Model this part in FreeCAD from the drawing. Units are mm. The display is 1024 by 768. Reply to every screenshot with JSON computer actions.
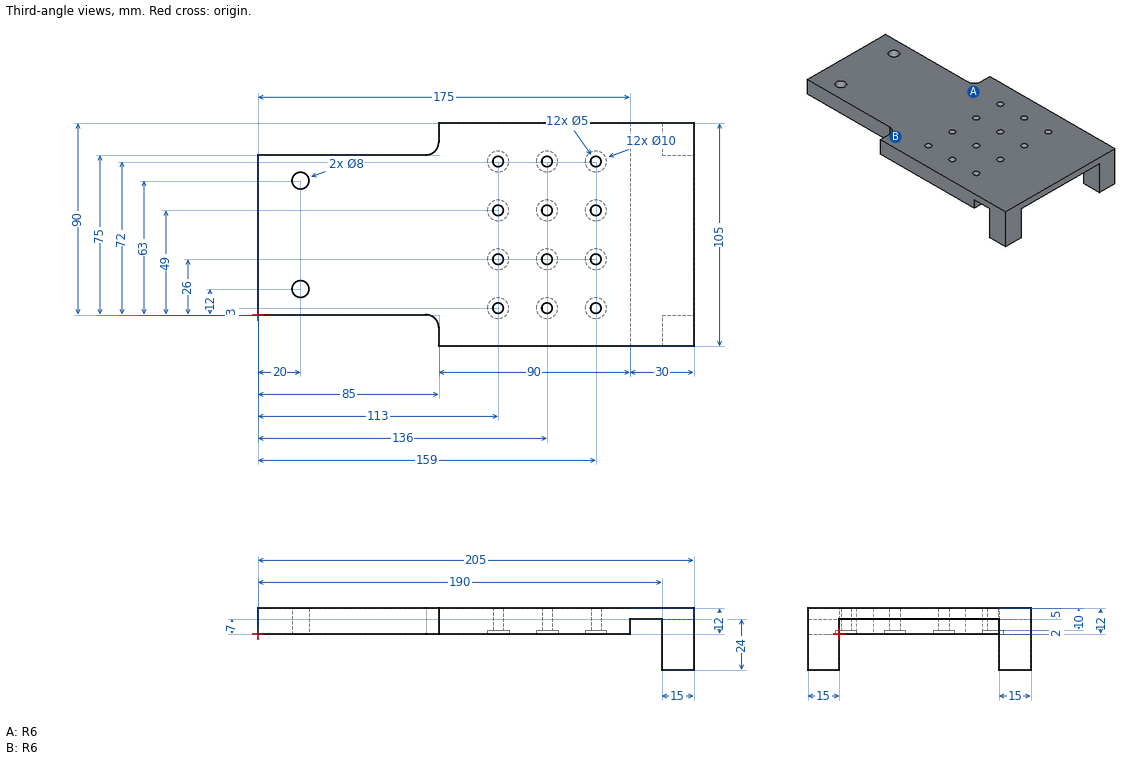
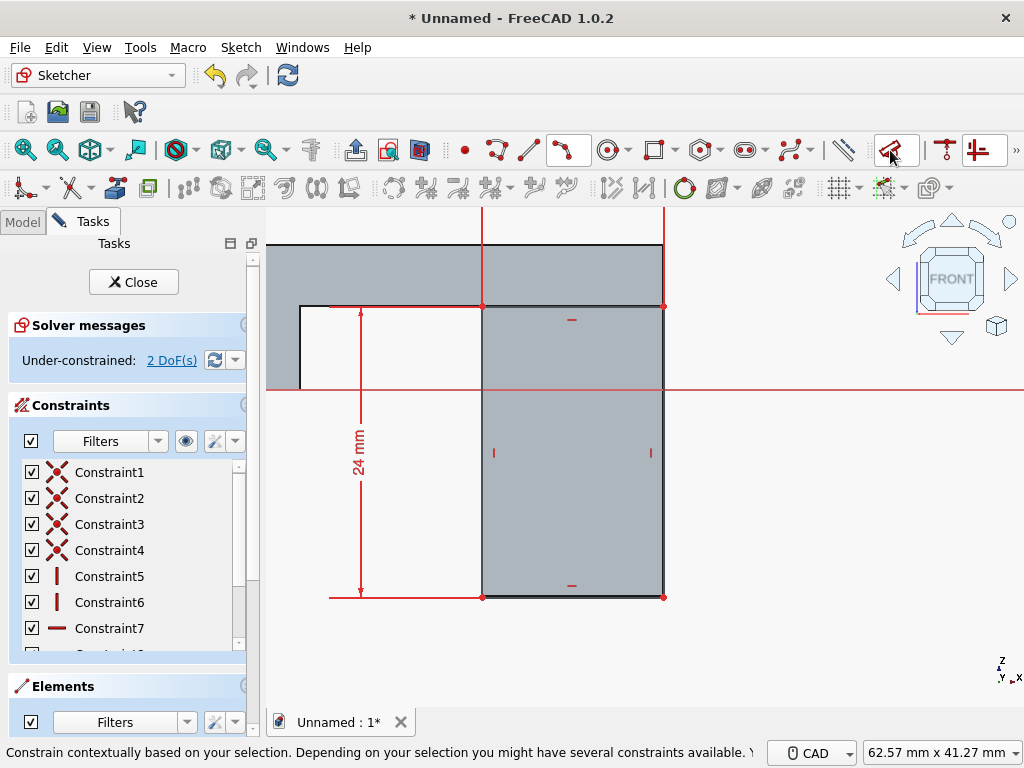
{"action": "left_click", "coordinate": [482, 307]}
{"action": "left_click", "coordinate": [516, 349]}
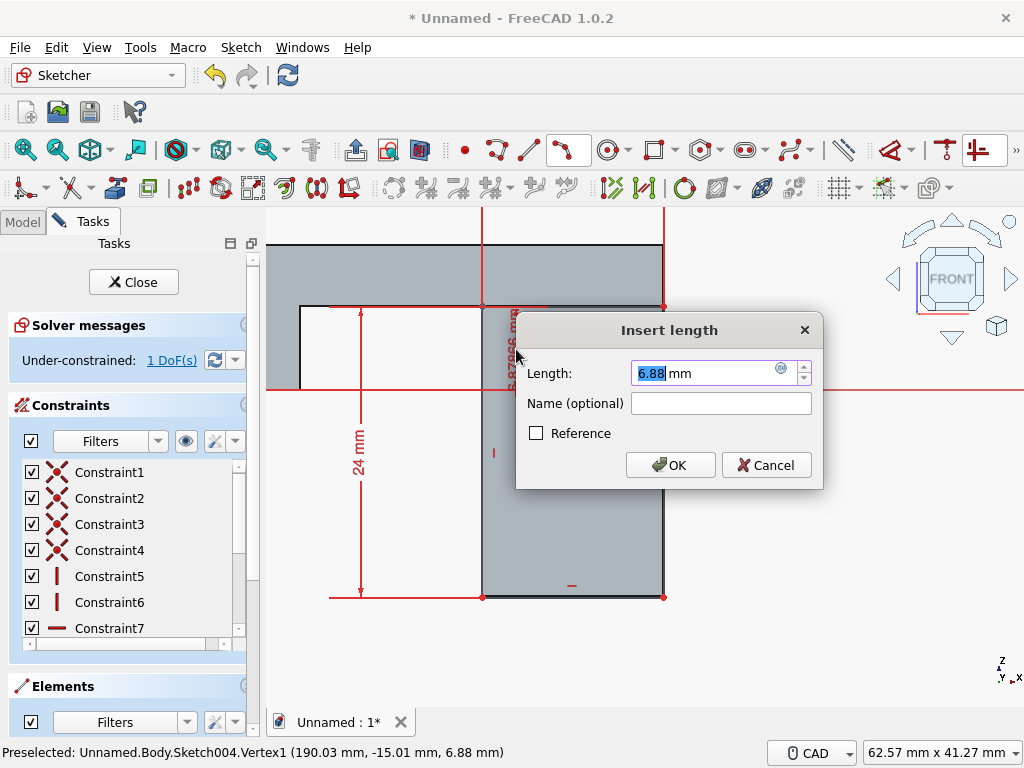
{"action": "type", "text": "7"}
{"action": "key", "text": "Return"}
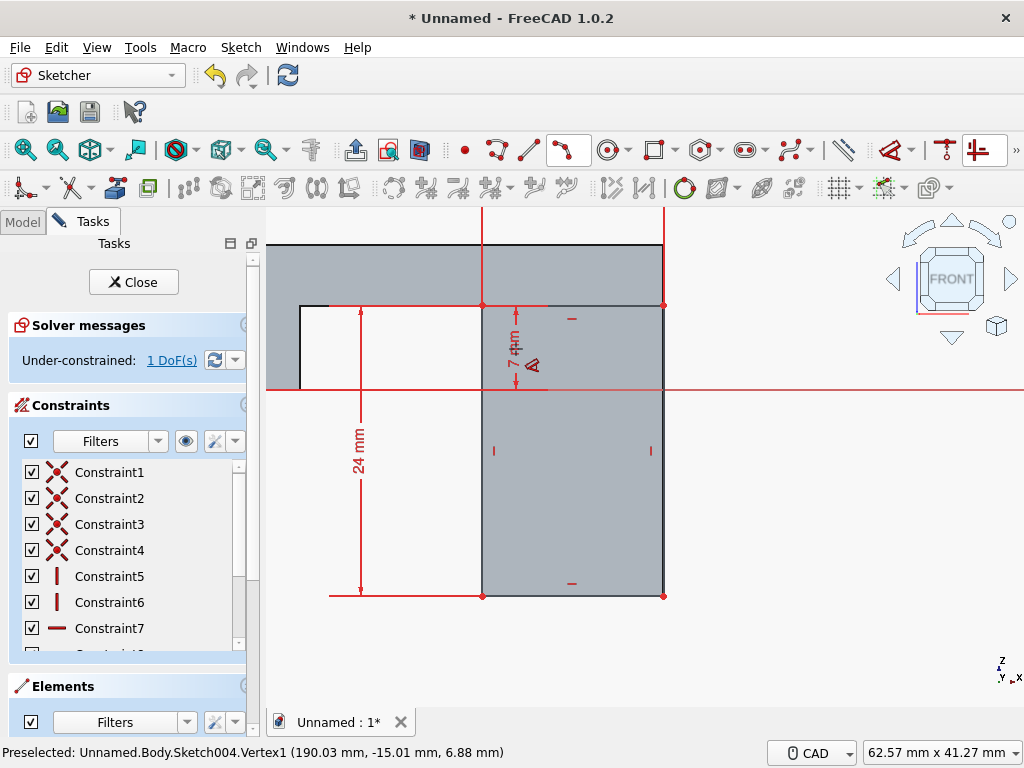
{"action": "left_click", "coordinate": [482, 306]}
{"action": "left_click", "coordinate": [388, 272]}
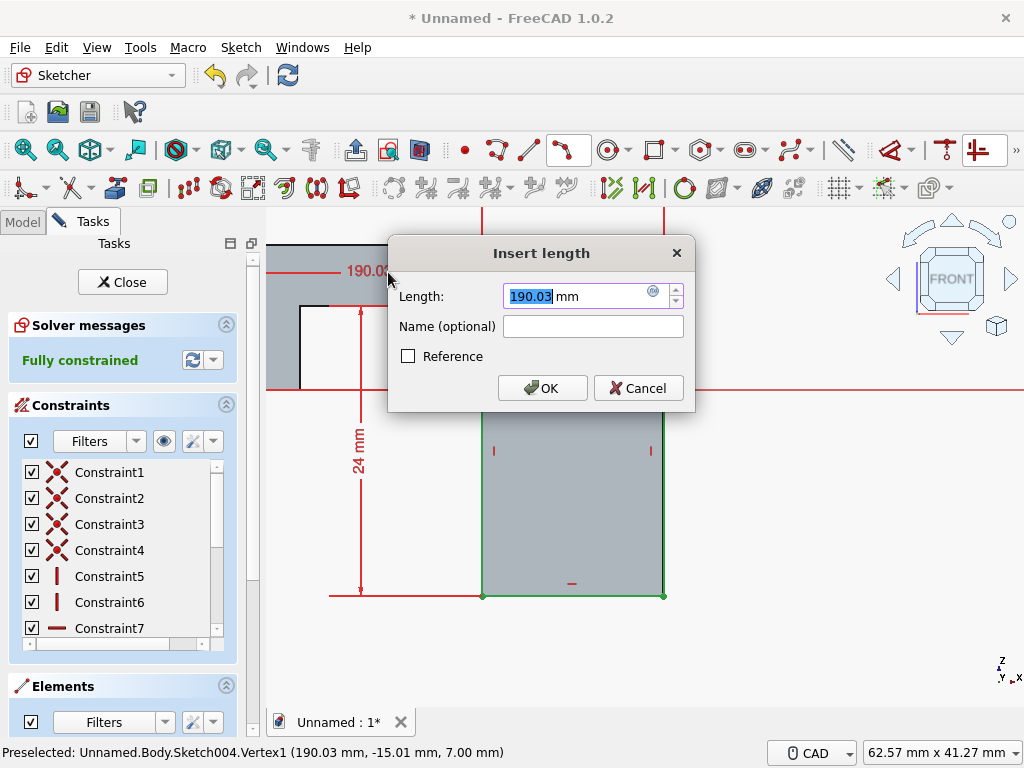
{"action": "type", "text": "190"}
{"action": "key", "text": "Return"}
{"action": "key", "text": "Escape"}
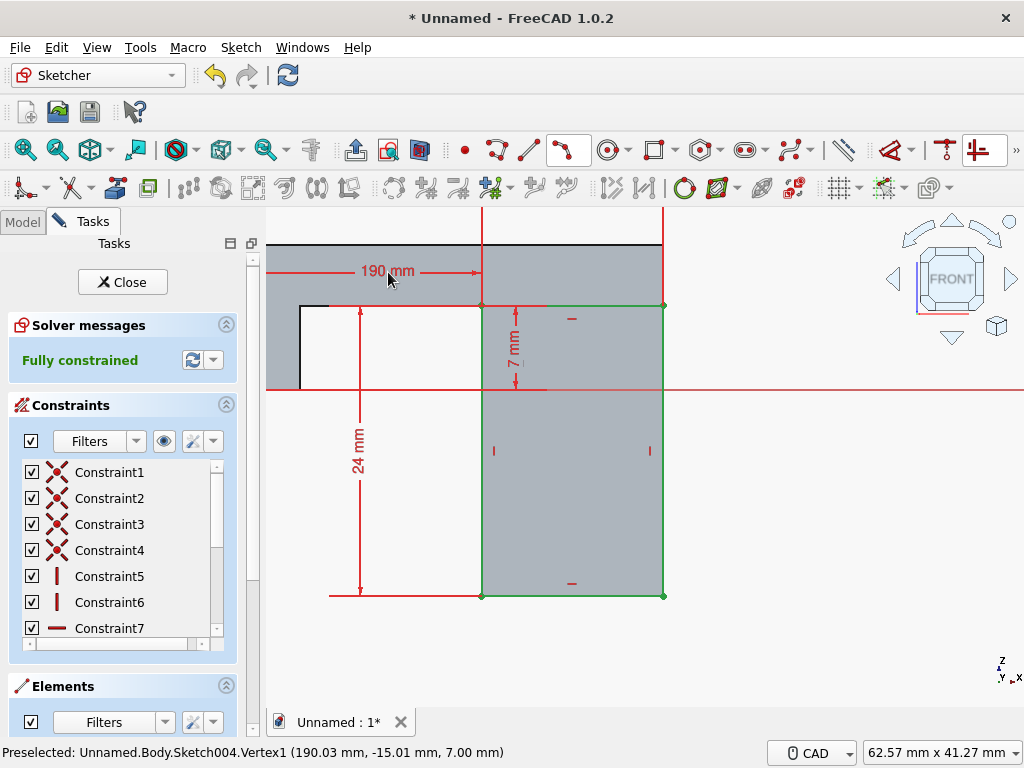
{"action": "left_click", "coordinate": [123, 282]}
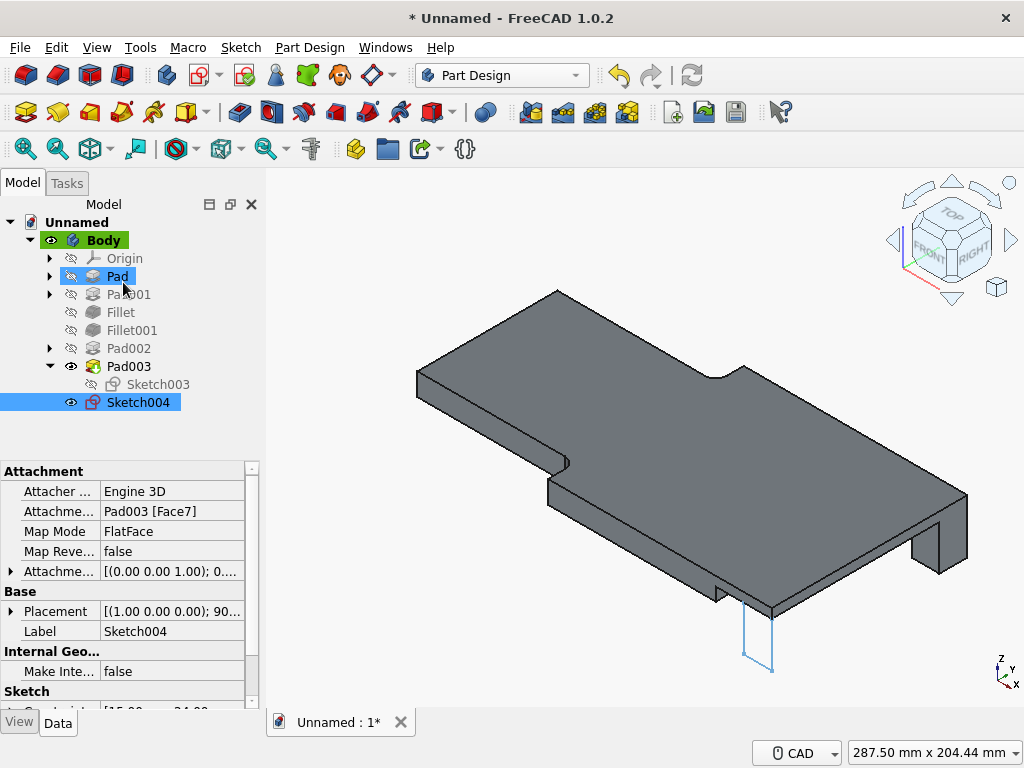
{"action": "left_click", "coordinate": [26, 112]}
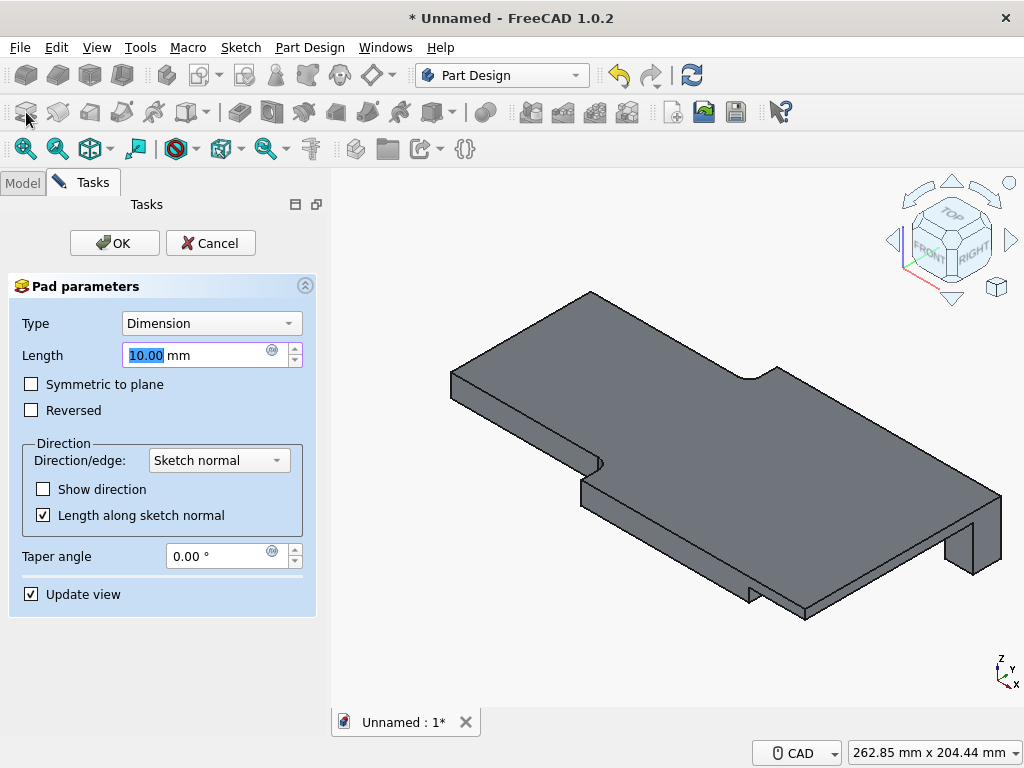
{"action": "type", "text": "15"}
{"action": "key", "text": "Tab"}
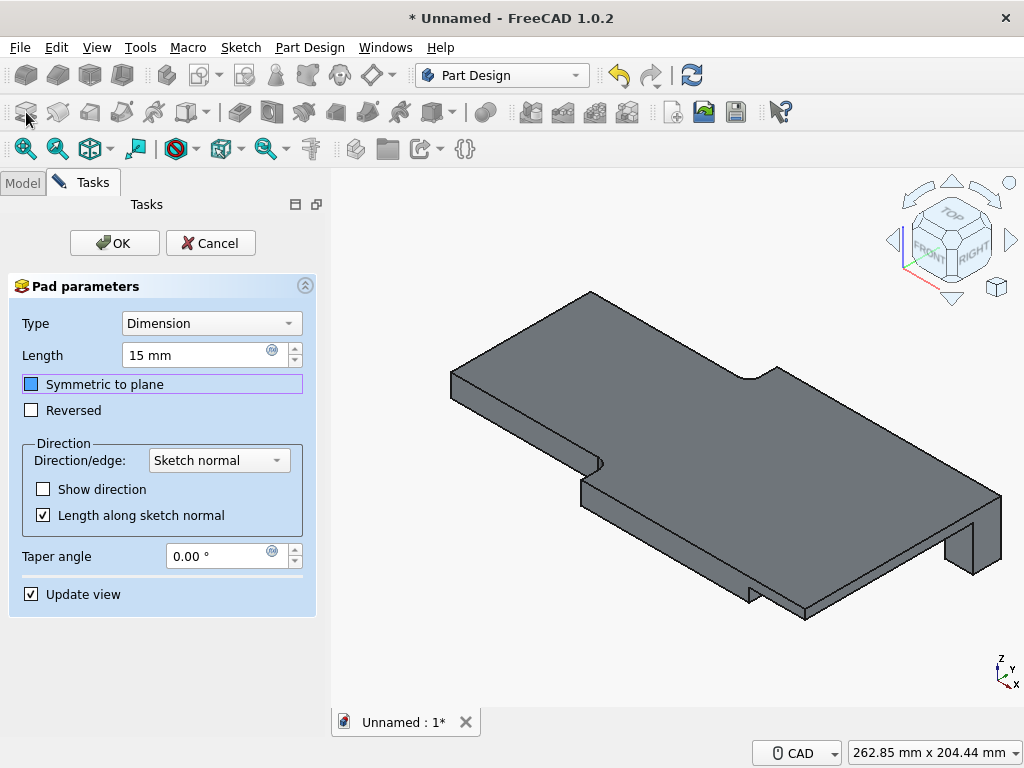
{"action": "left_click", "coordinate": [30, 410]}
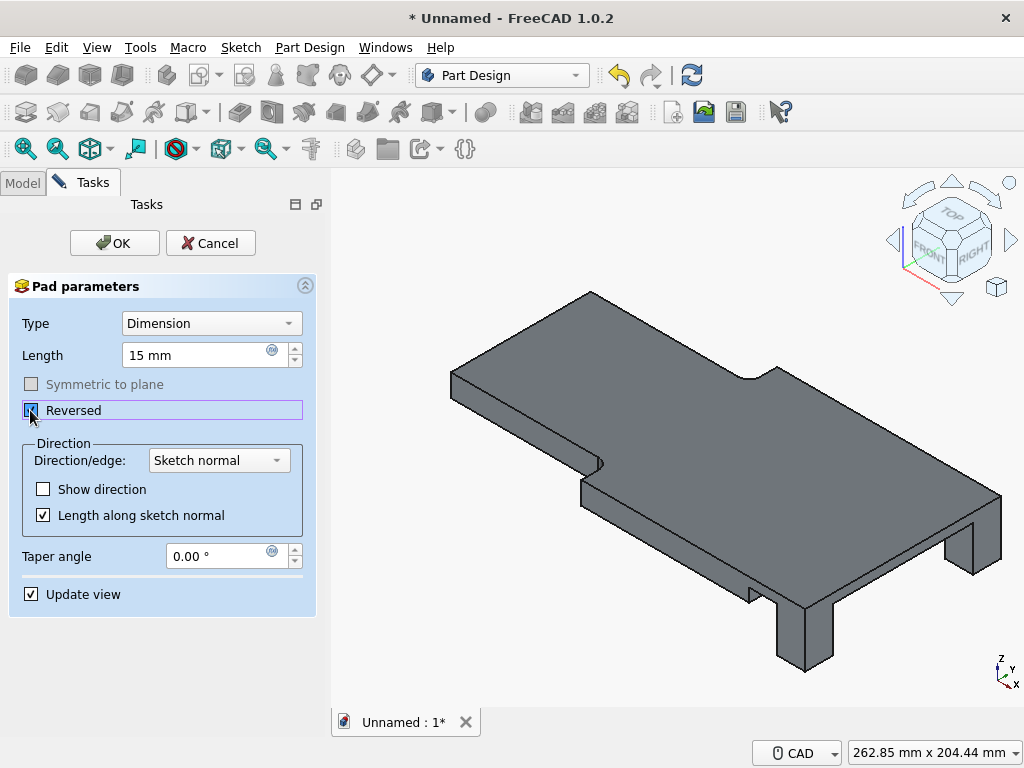
{"action": "left_click", "coordinate": [115, 243]}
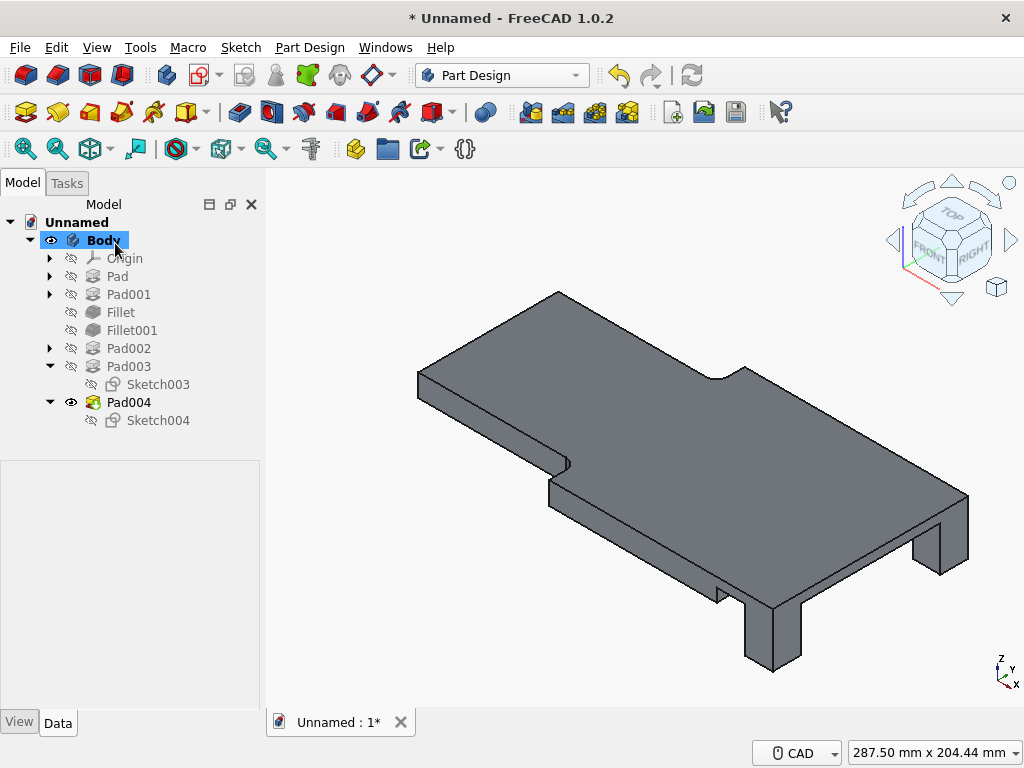
{"action": "left_click", "coordinate": [200, 76]}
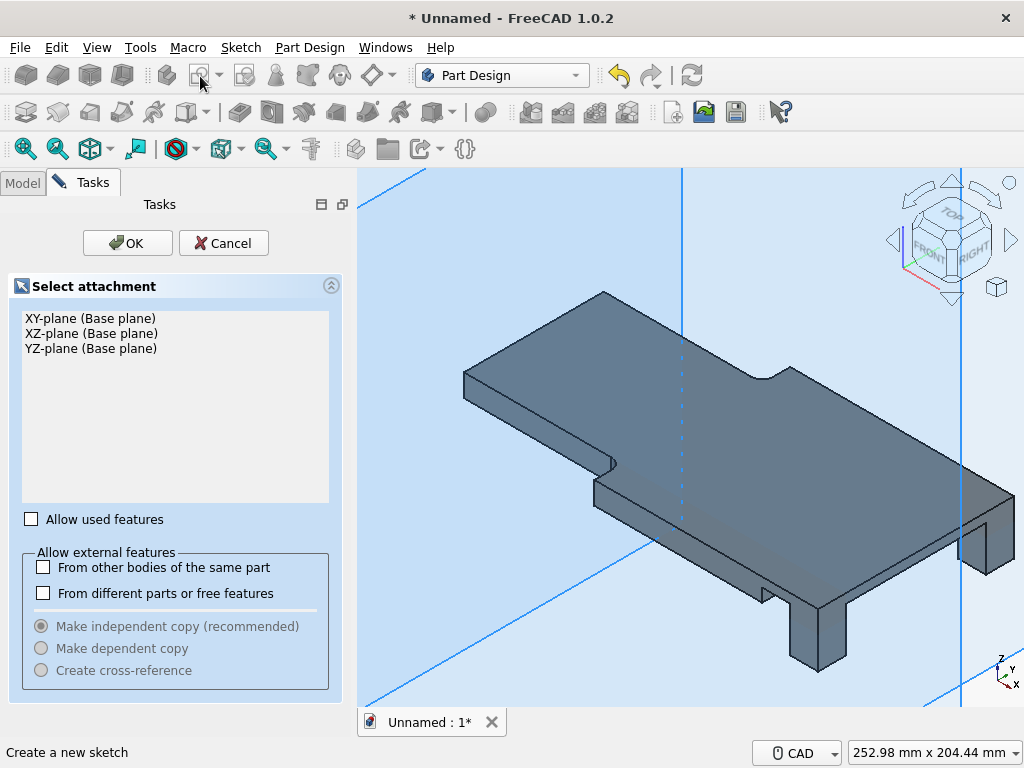
{"action": "left_click", "coordinate": [82, 318]}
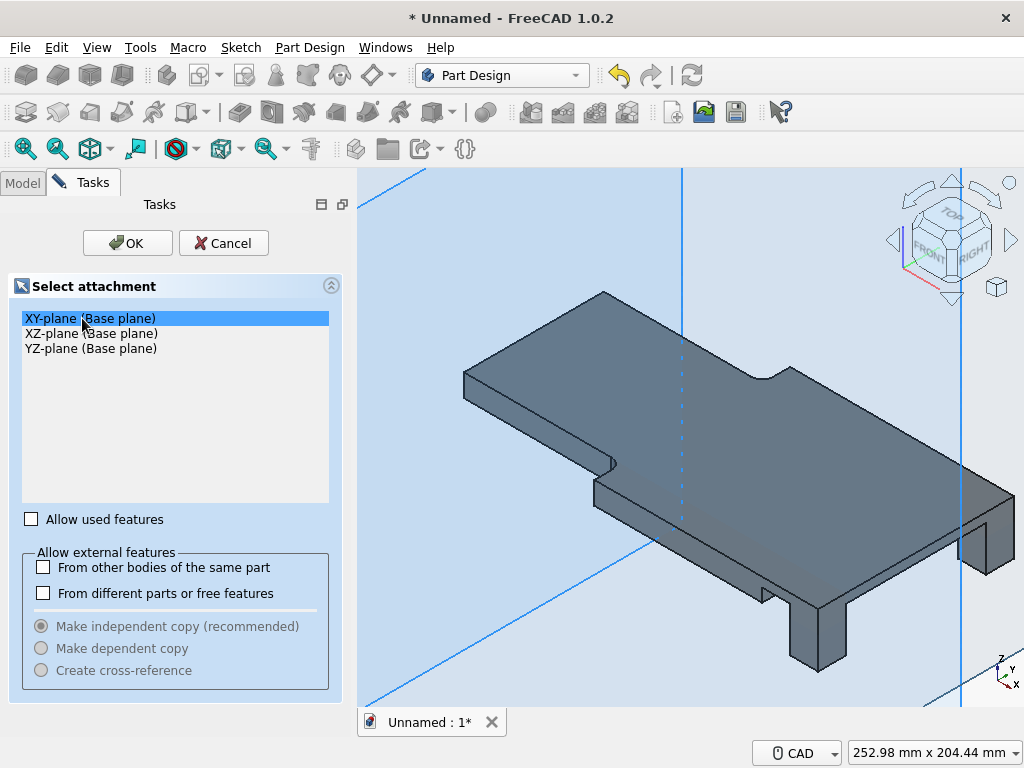
{"action": "left_click", "coordinate": [128, 243]}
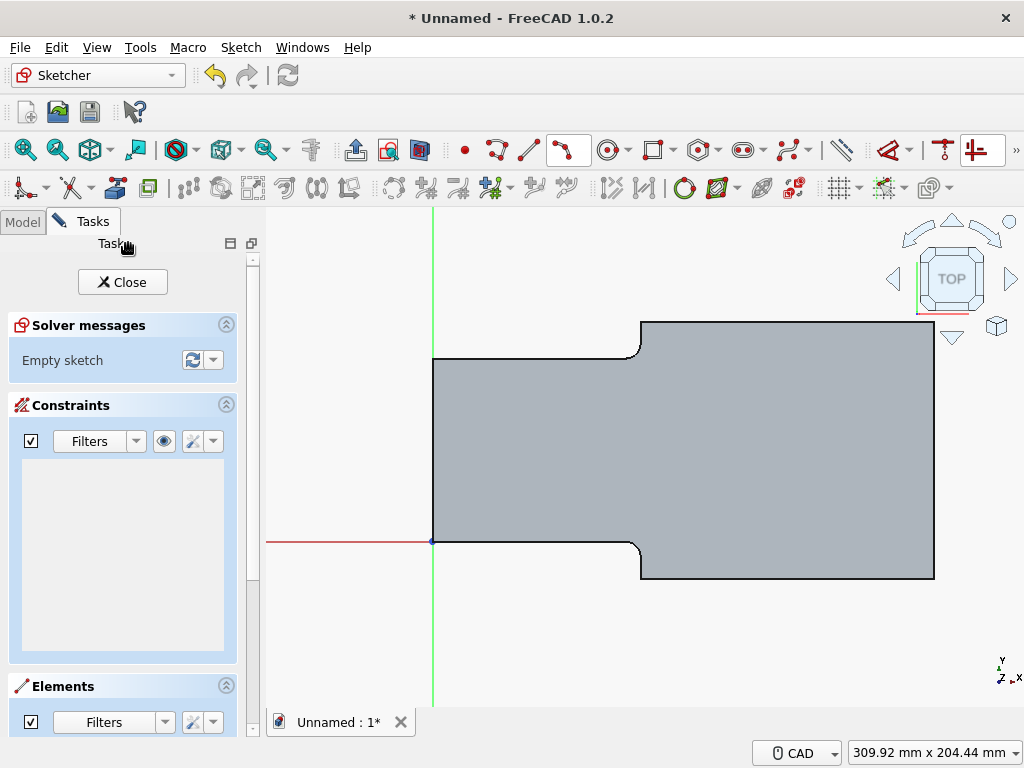
{"action": "left_click", "coordinate": [420, 150]}